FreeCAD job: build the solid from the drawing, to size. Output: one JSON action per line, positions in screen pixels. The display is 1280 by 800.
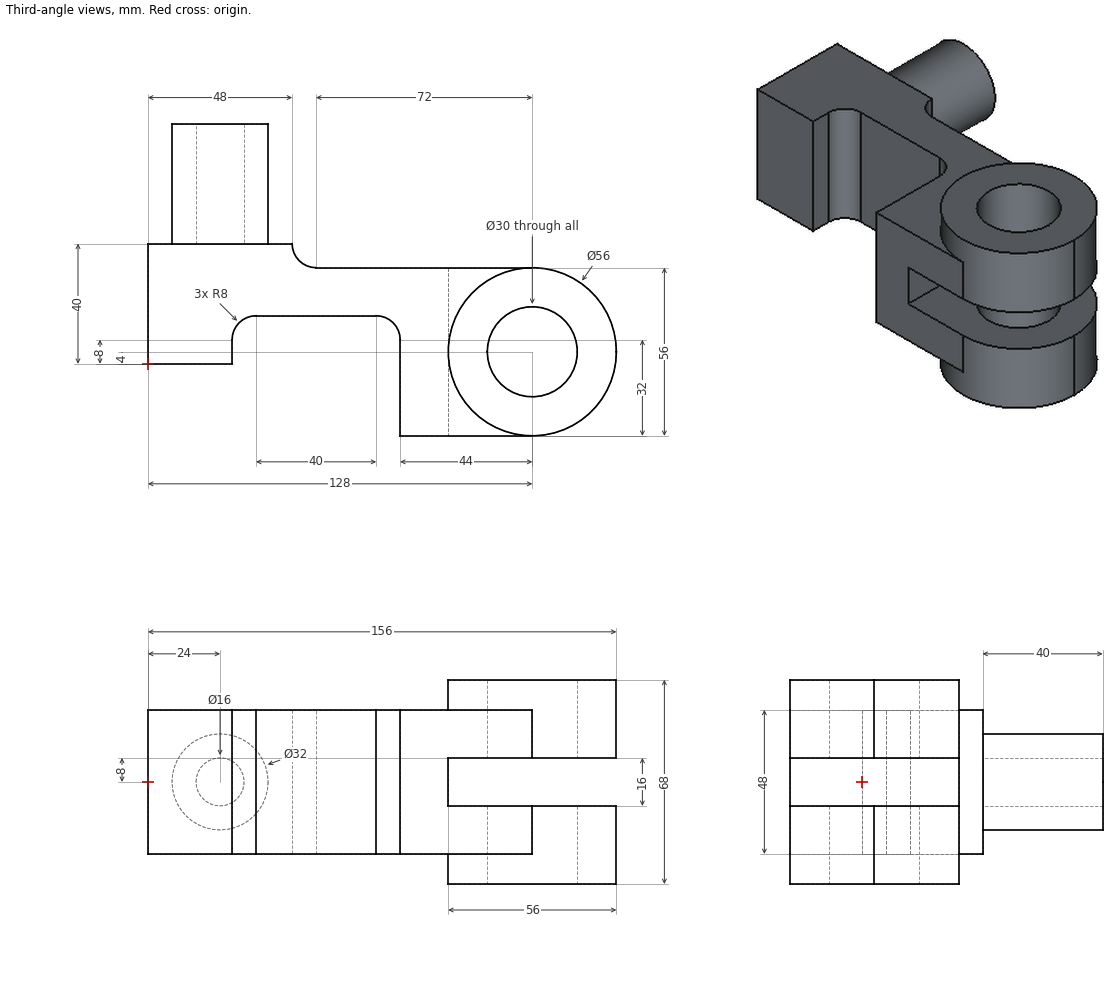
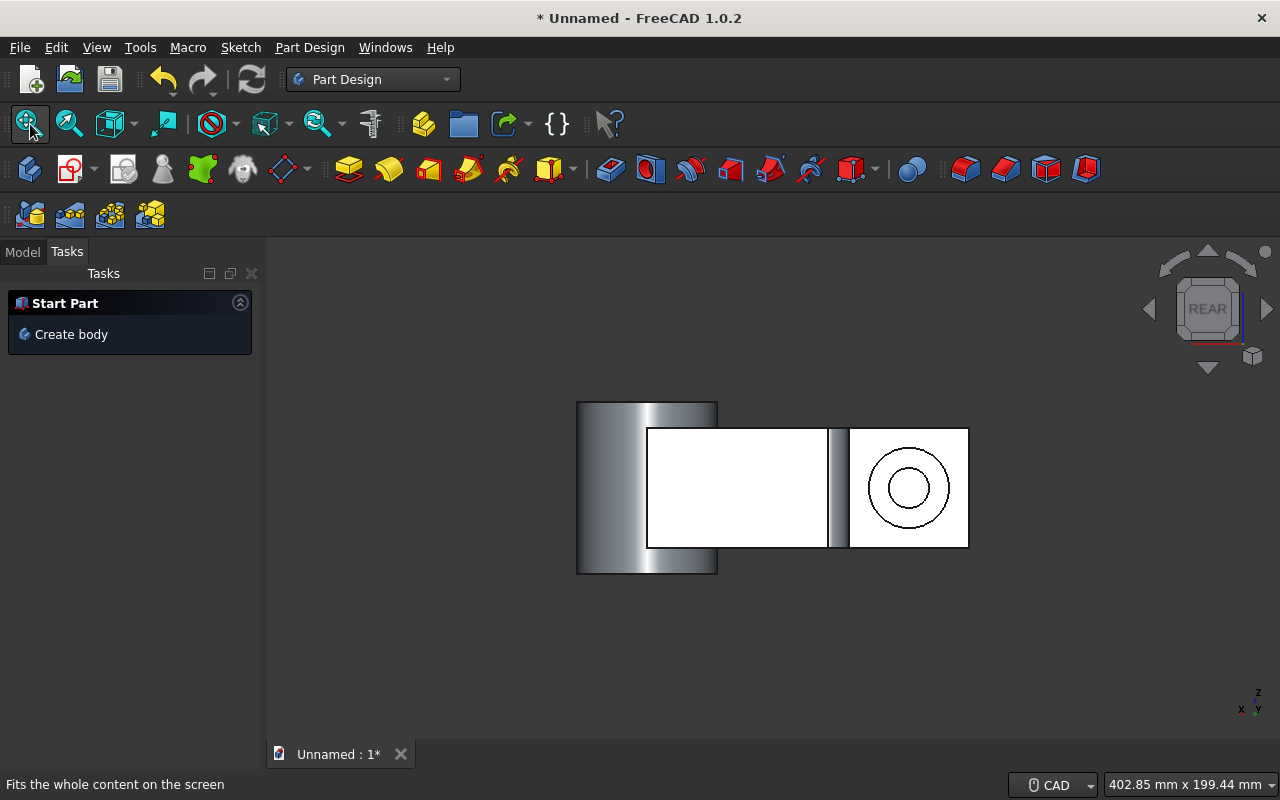
{"action": "left_click", "coordinate": [712, 487]}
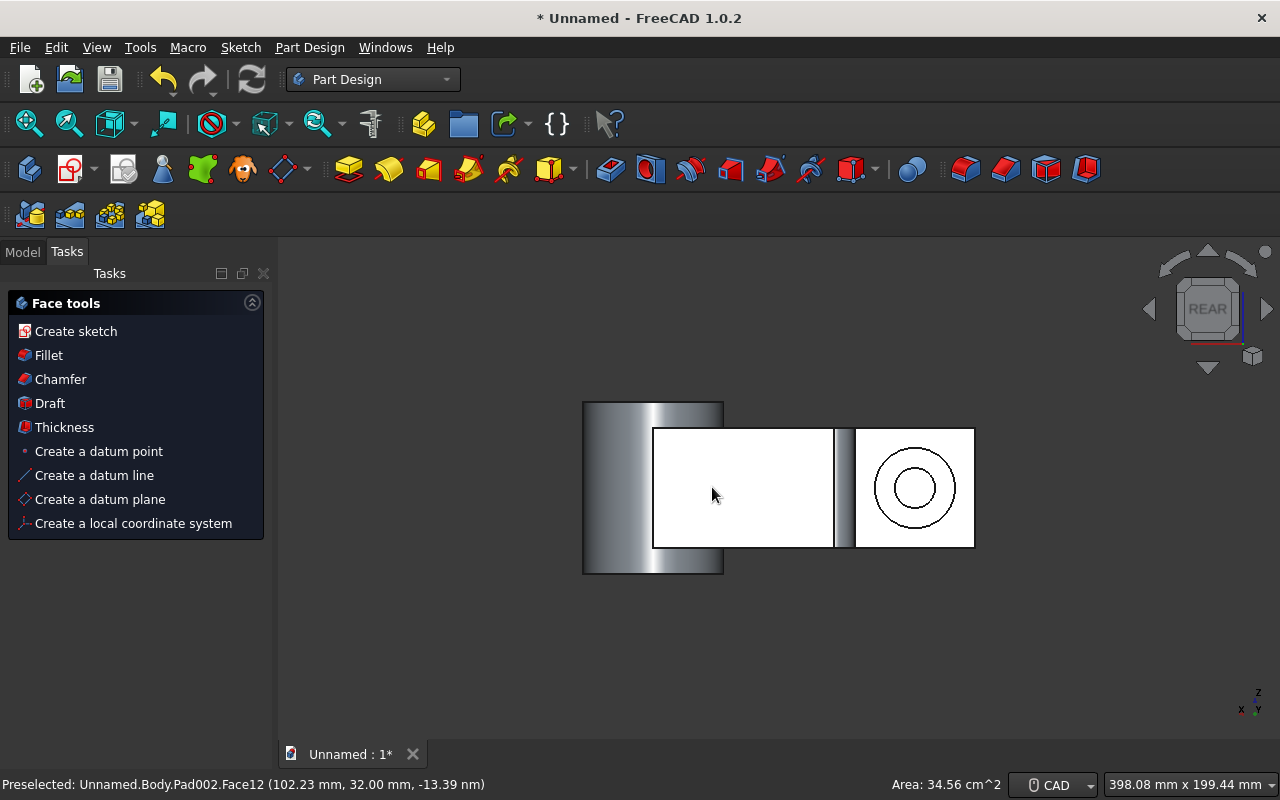
{"action": "left_click", "coordinate": [70, 170]}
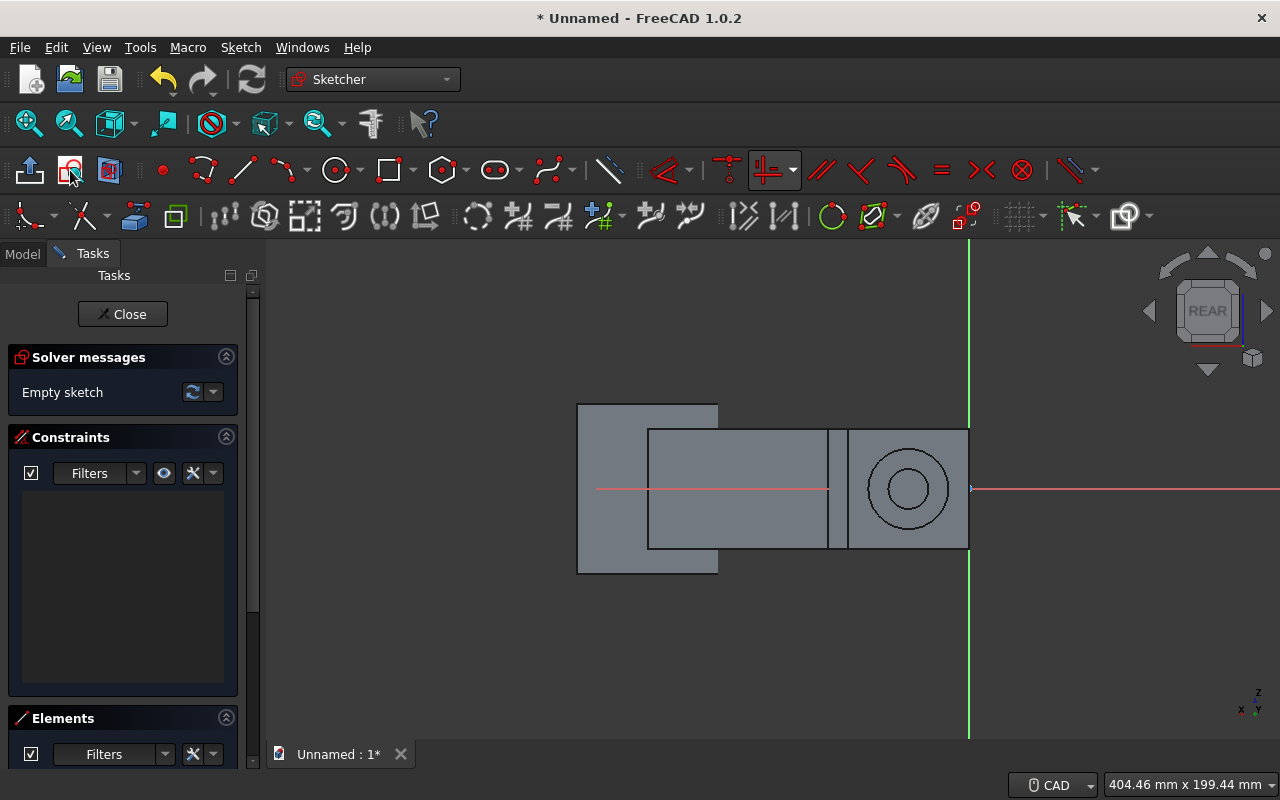
{"action": "scroll", "coordinate": [629, 489], "scroll_direction": "up", "scroll_amount": 7}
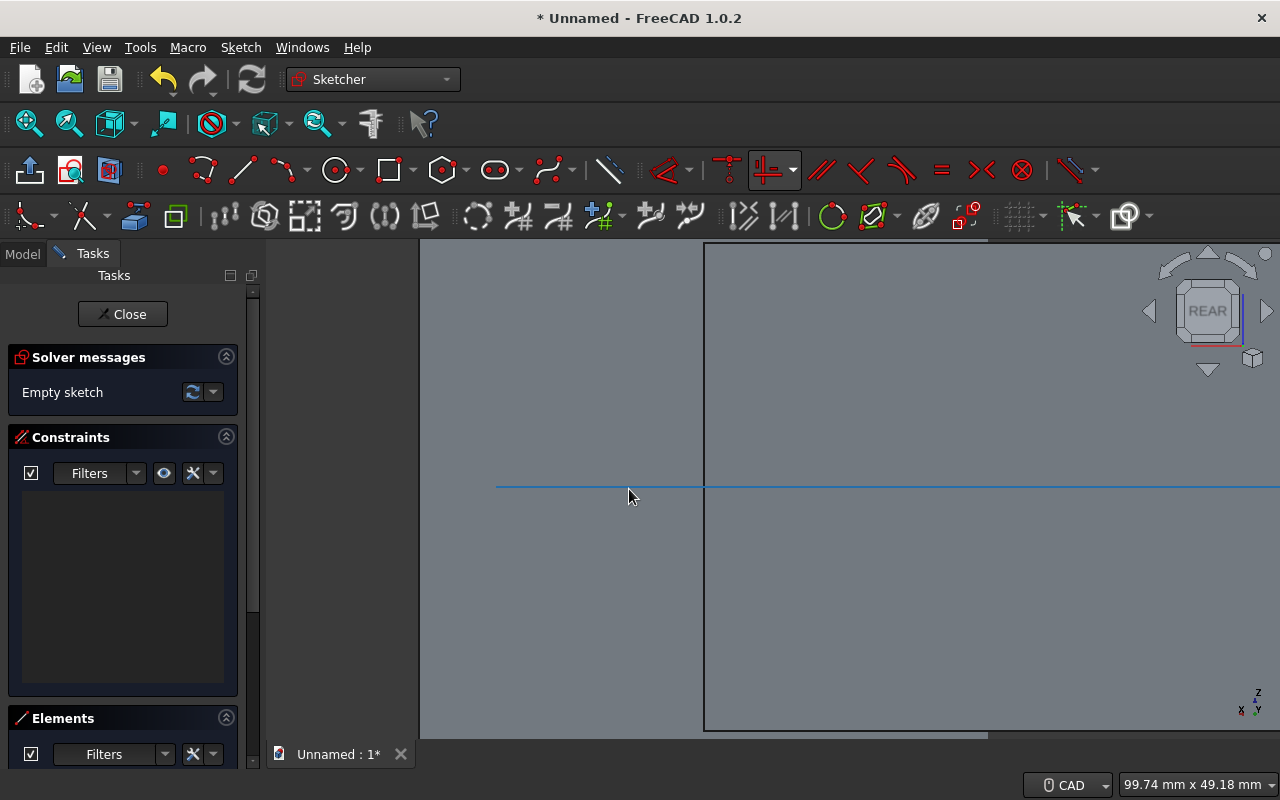
{"action": "key", "text": "g r"}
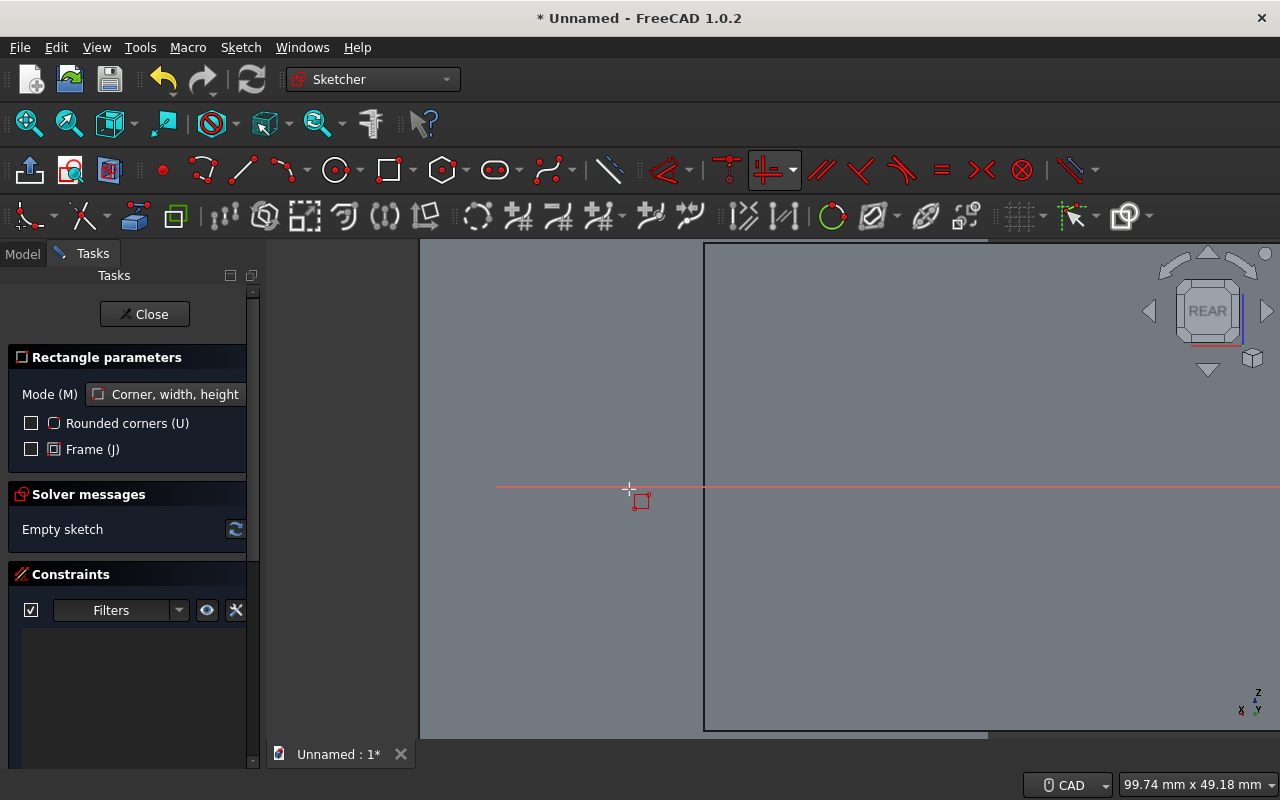
{"action": "left_click", "coordinate": [419, 406]}
{"action": "mouse_move", "coordinate": [988, 569]}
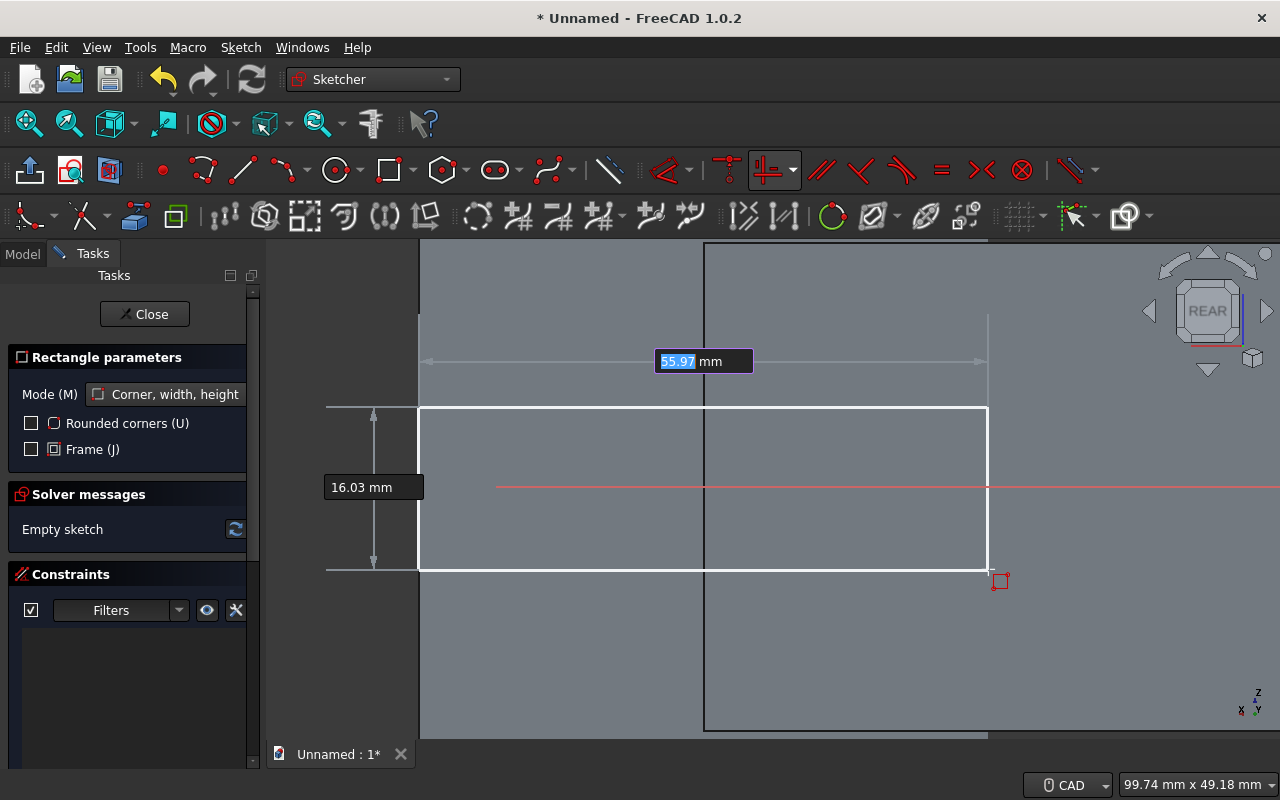
{"action": "type", "text": "56"}
{"action": "key", "text": "Tab"}
{"action": "type", "text": "16"}
{"action": "key", "text": "Return"}
{"action": "key", "text": "Escape"}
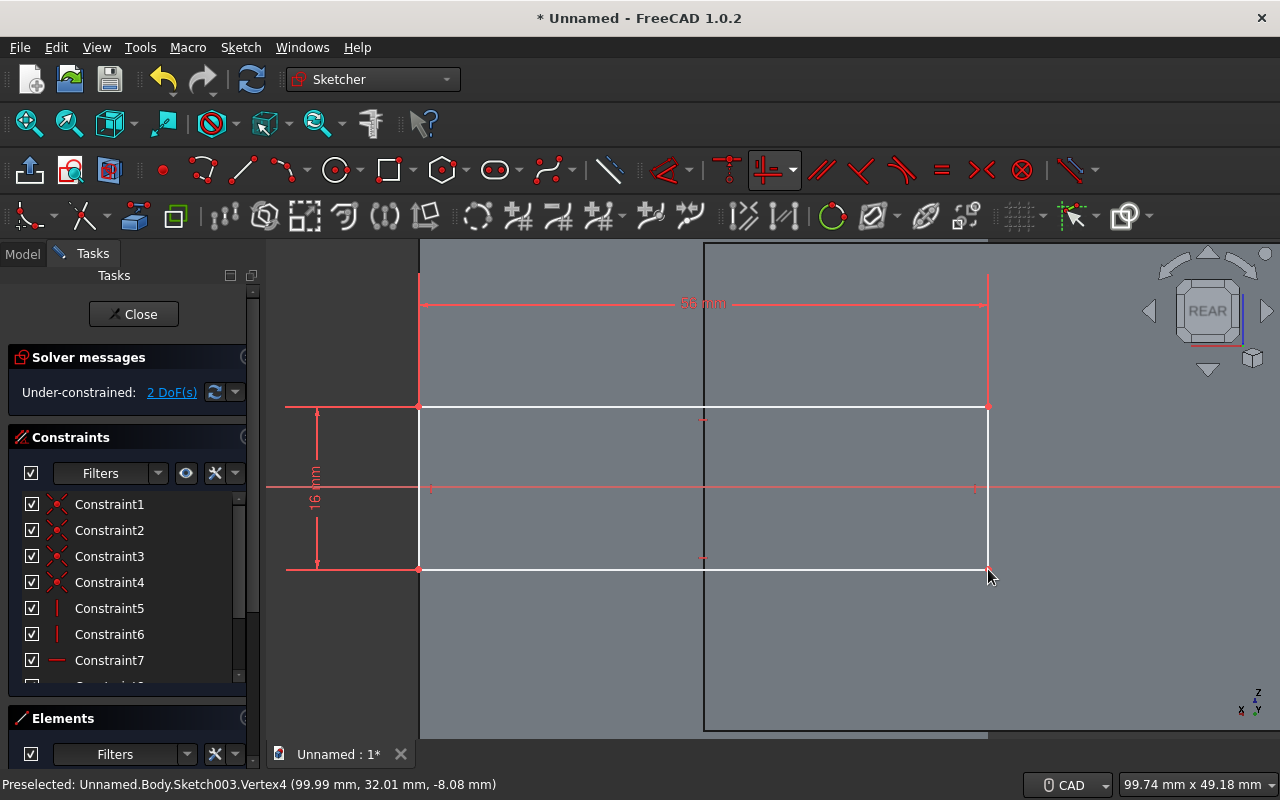
{"action": "key", "text": "d"}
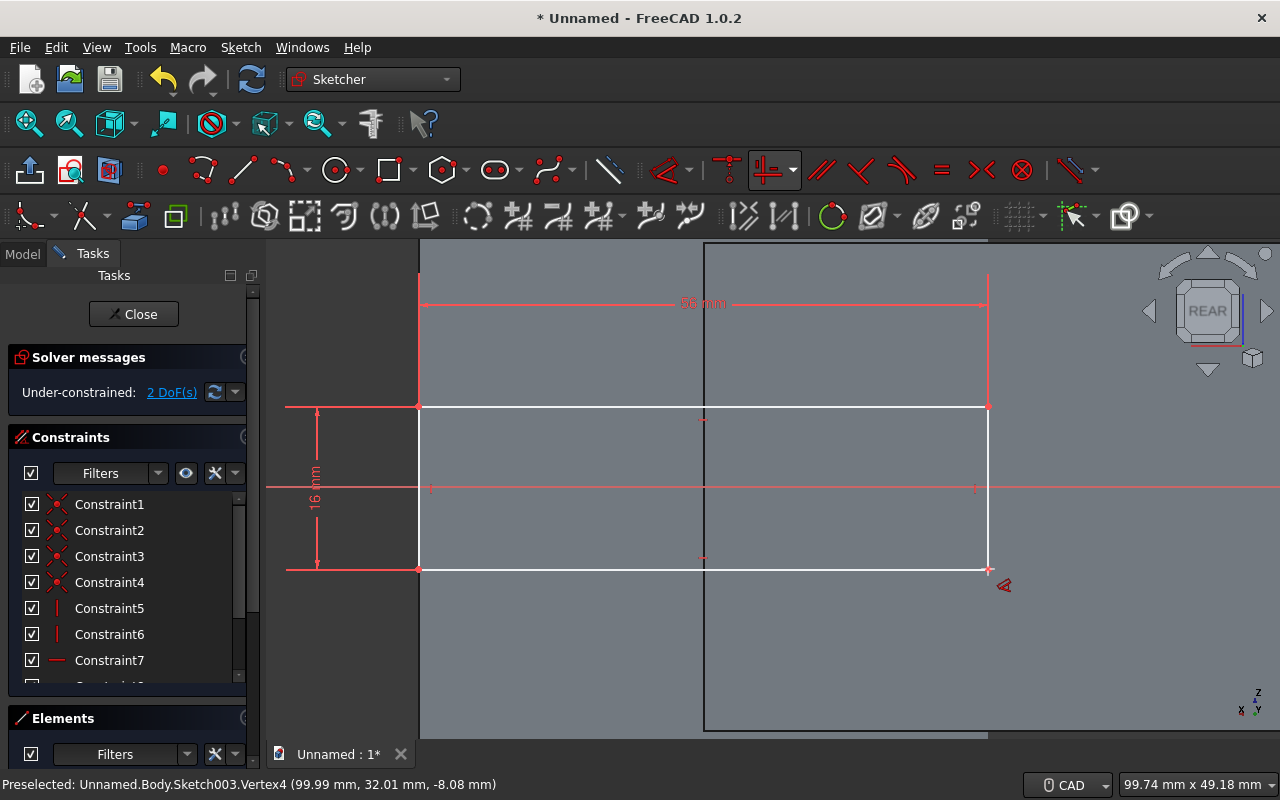
{"action": "left_click", "coordinate": [419, 407]}
{"action": "left_click", "coordinate": [385, 447]}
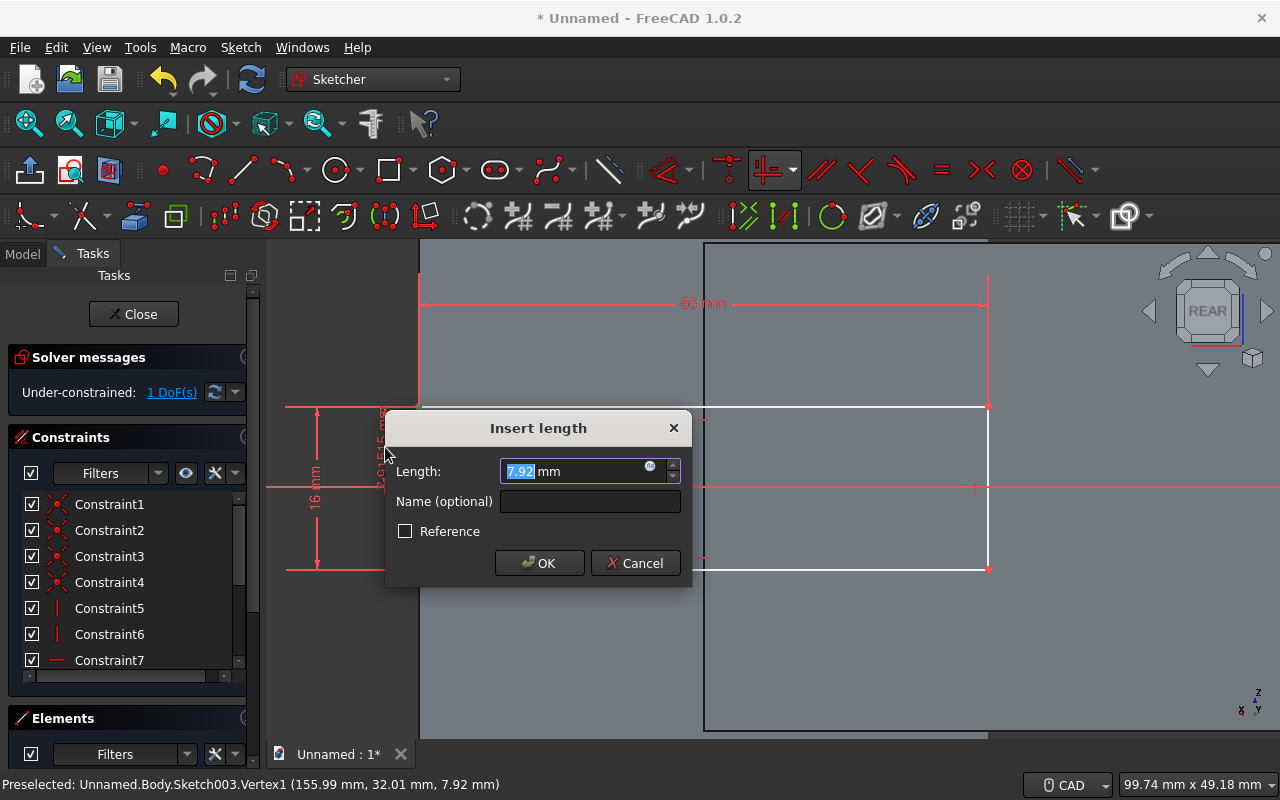
{"action": "type", "text": "8"}
{"action": "key", "text": "Return"}